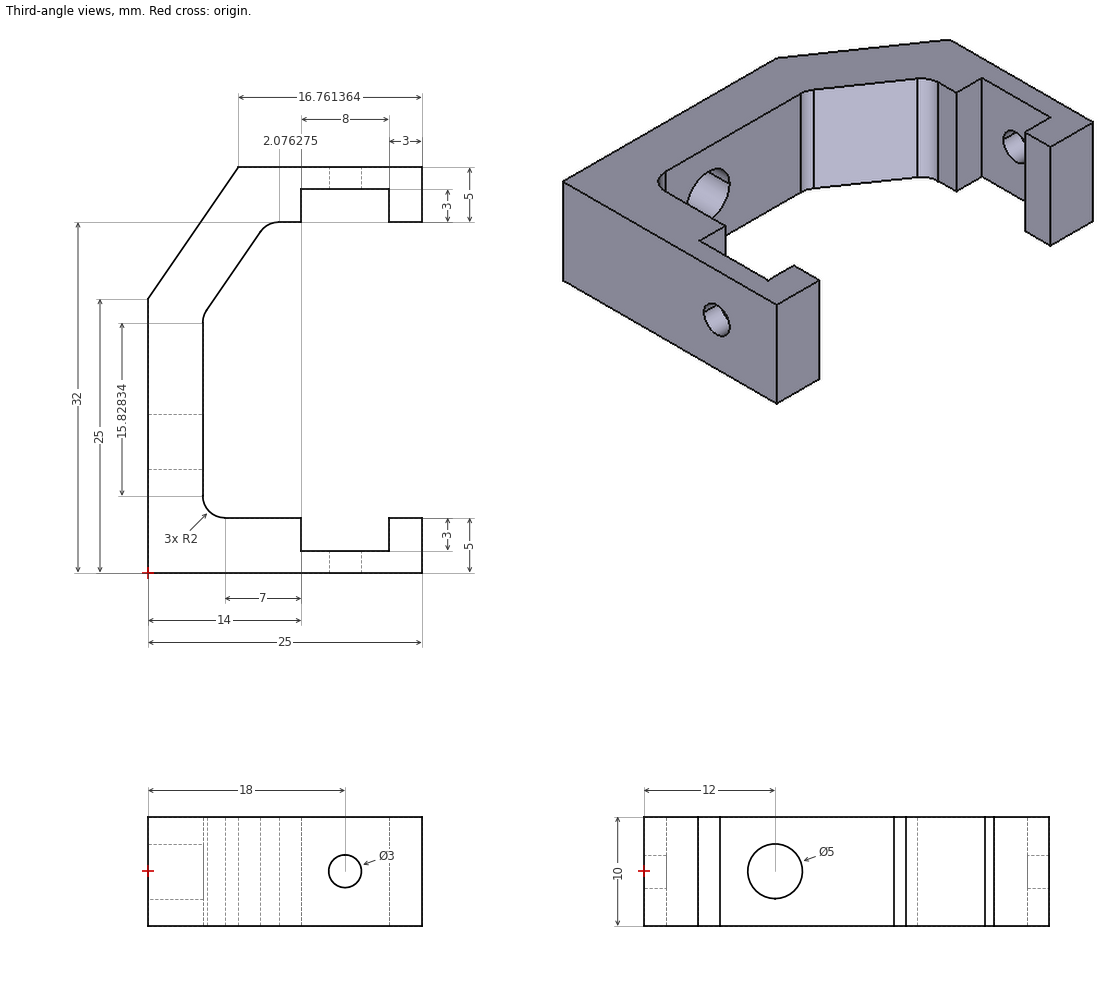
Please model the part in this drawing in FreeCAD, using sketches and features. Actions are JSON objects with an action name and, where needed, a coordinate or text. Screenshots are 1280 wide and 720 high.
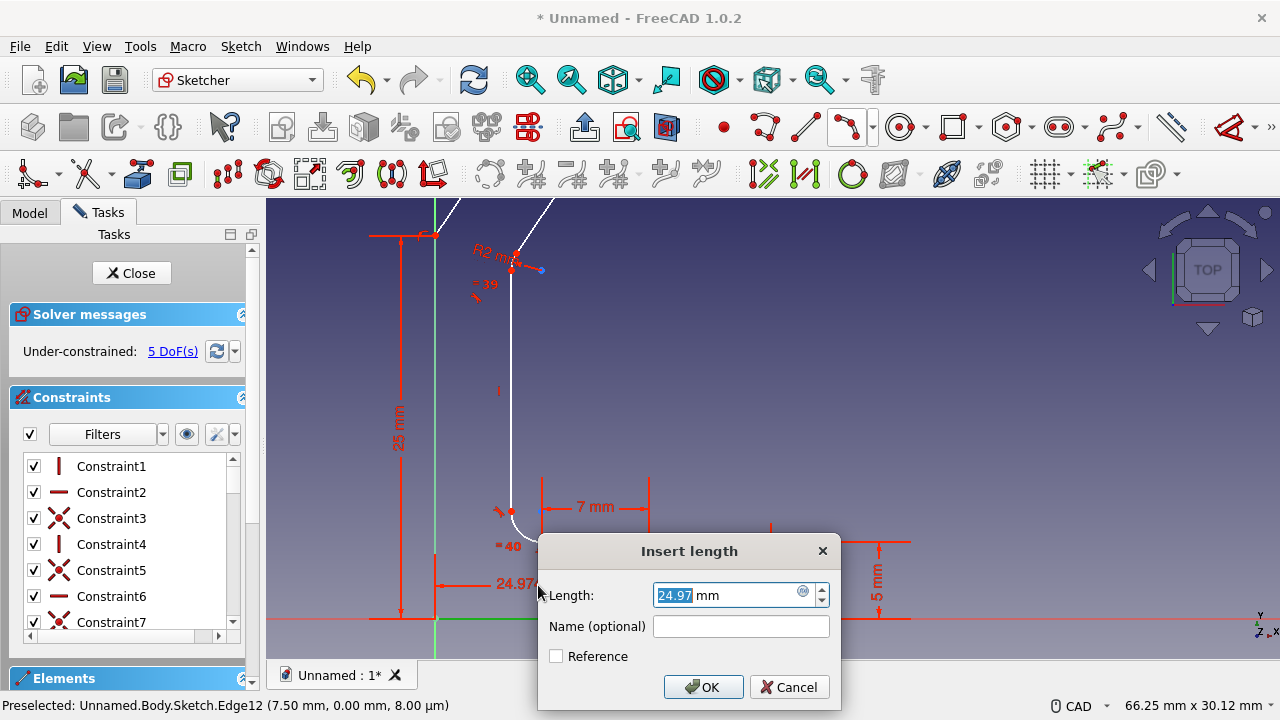
{"action": "type", "text": "25"}
{"action": "key", "text": "Return"}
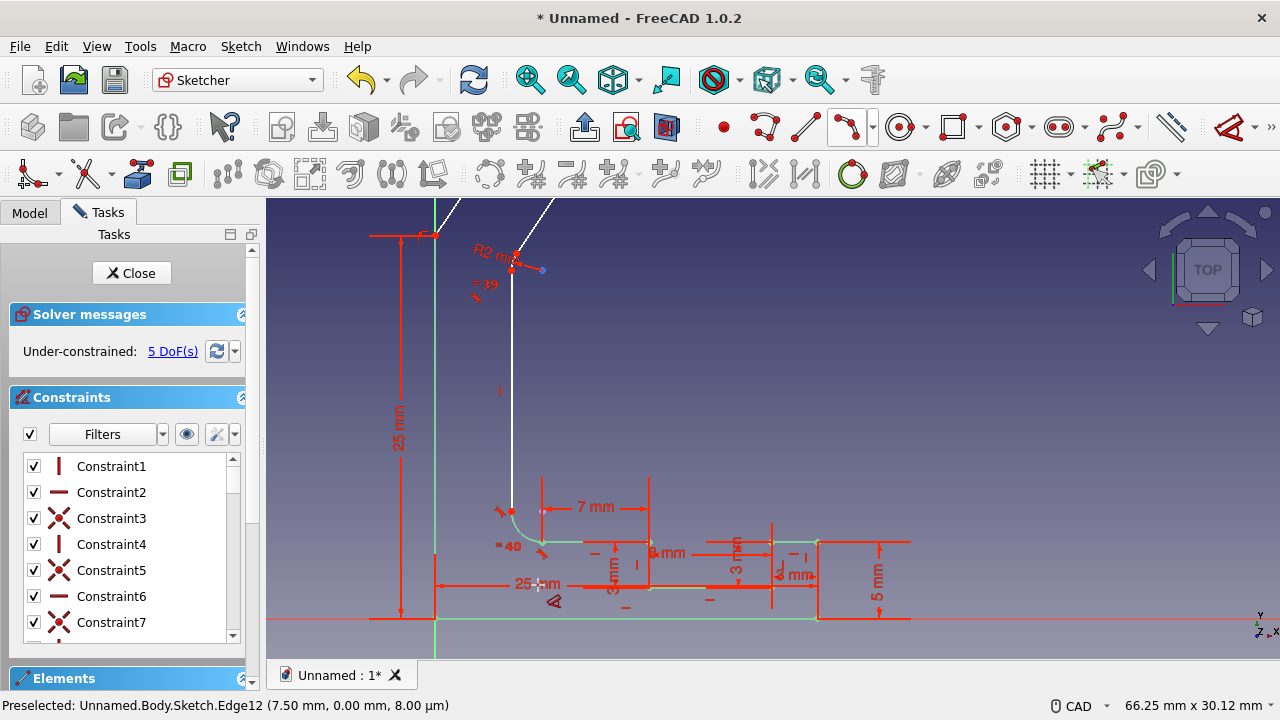
{"action": "scroll", "coordinate": [799, 542], "scroll_direction": "down", "scroll_amount": 3}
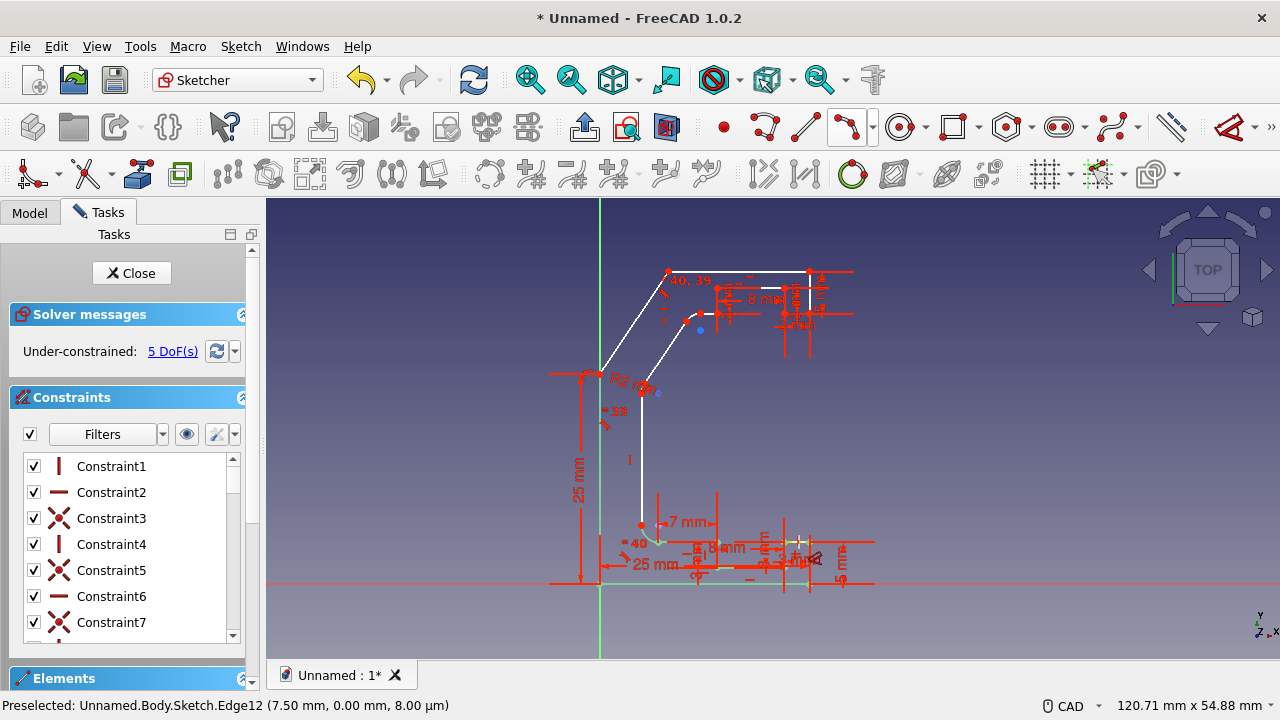
{"action": "left_click", "coordinate": [701, 314]}
{"action": "left_click", "coordinate": [566, 449]}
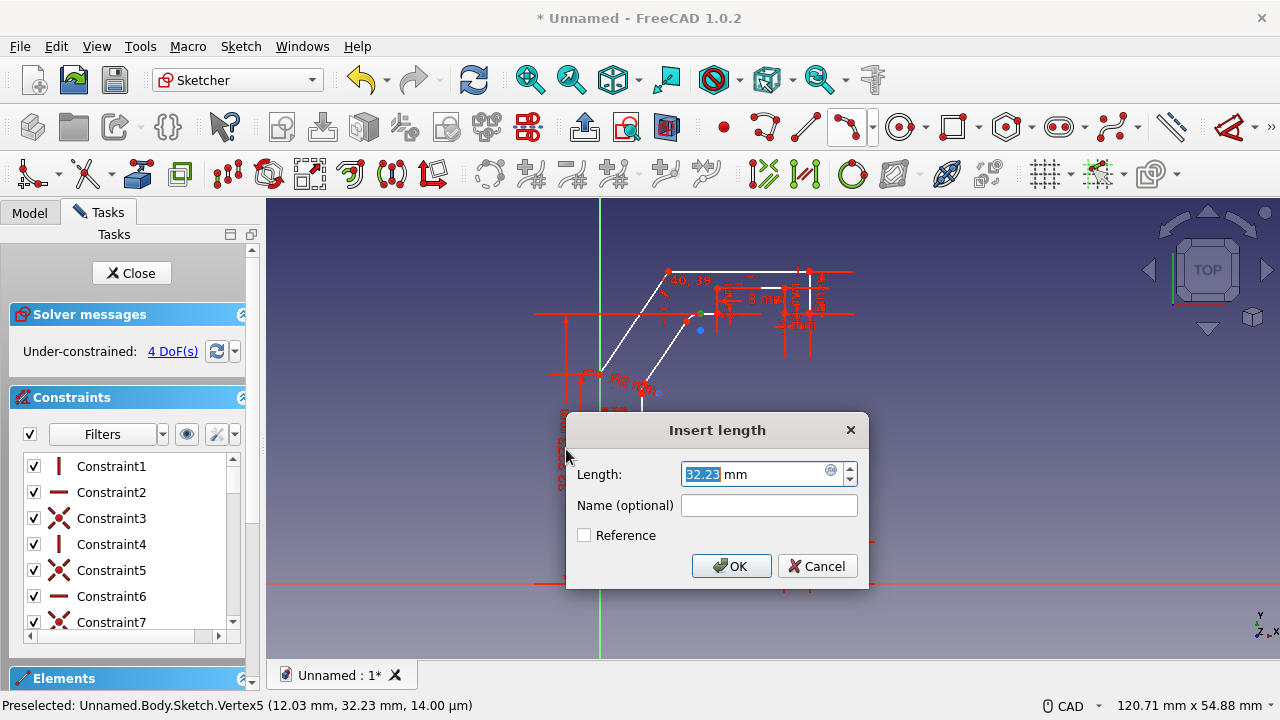
{"action": "type", "text": "32"}
{"action": "key", "text": "Return"}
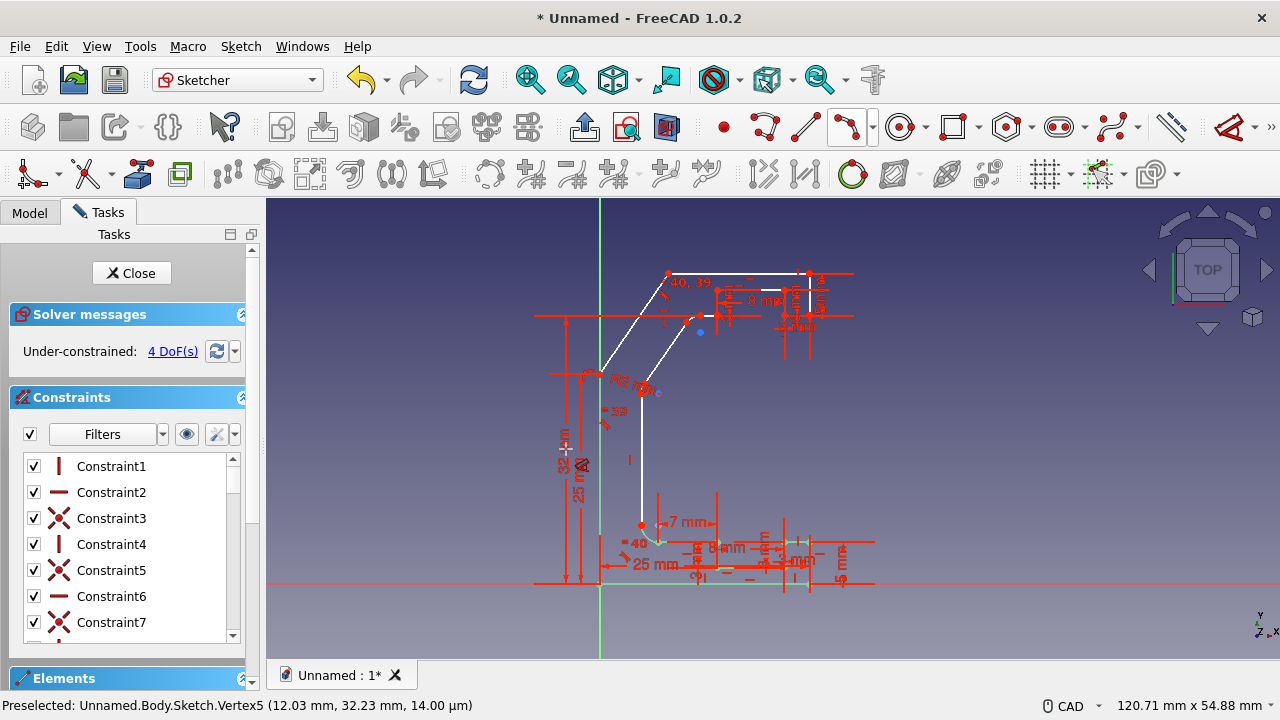
{"action": "left_click", "coordinate": [717, 316]}
{"action": "left_click", "coordinate": [658, 618]}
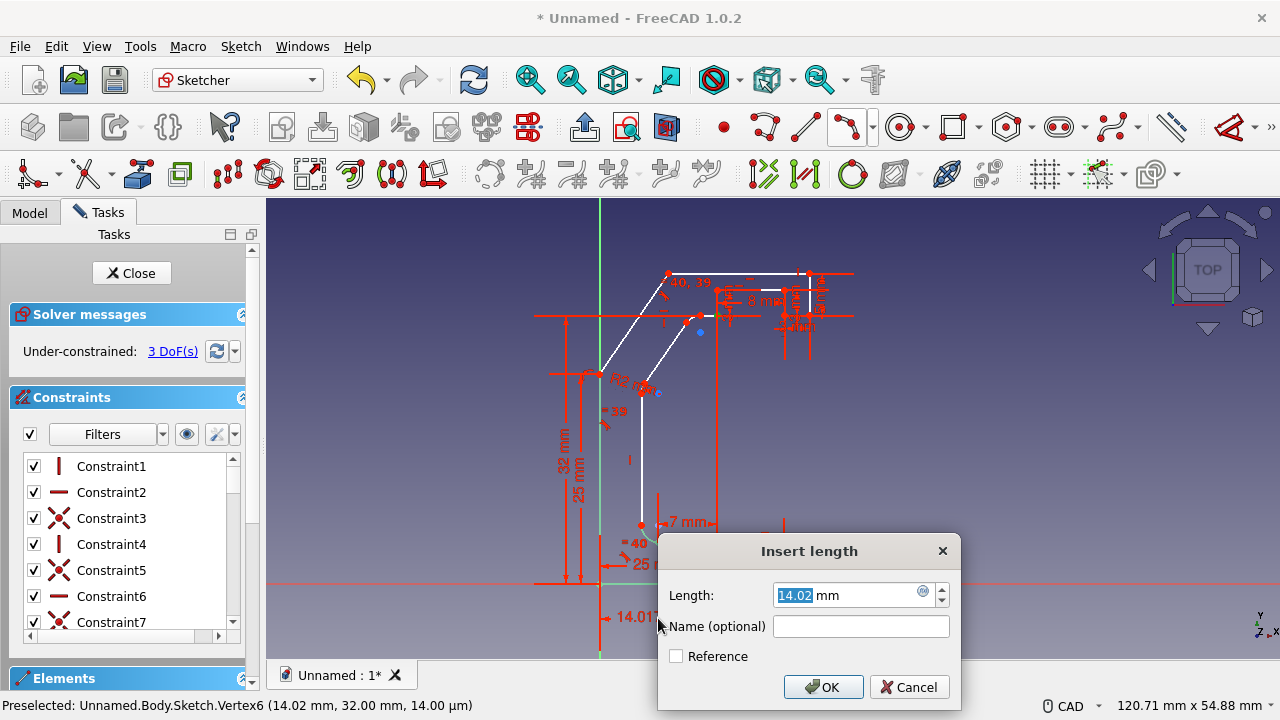
{"action": "type", "text": "14"}
{"action": "key", "text": "Return"}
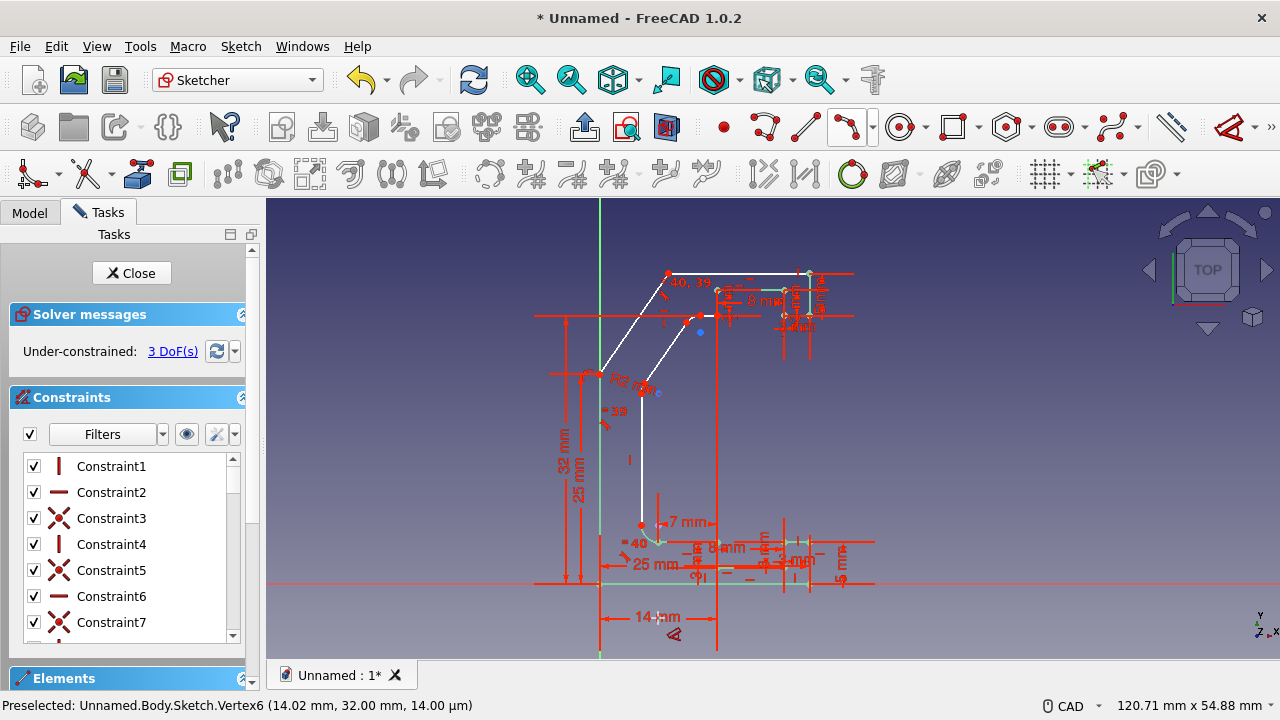
{"action": "left_click", "coordinate": [642, 486]}
{"action": "left_click", "coordinate": [676, 460]}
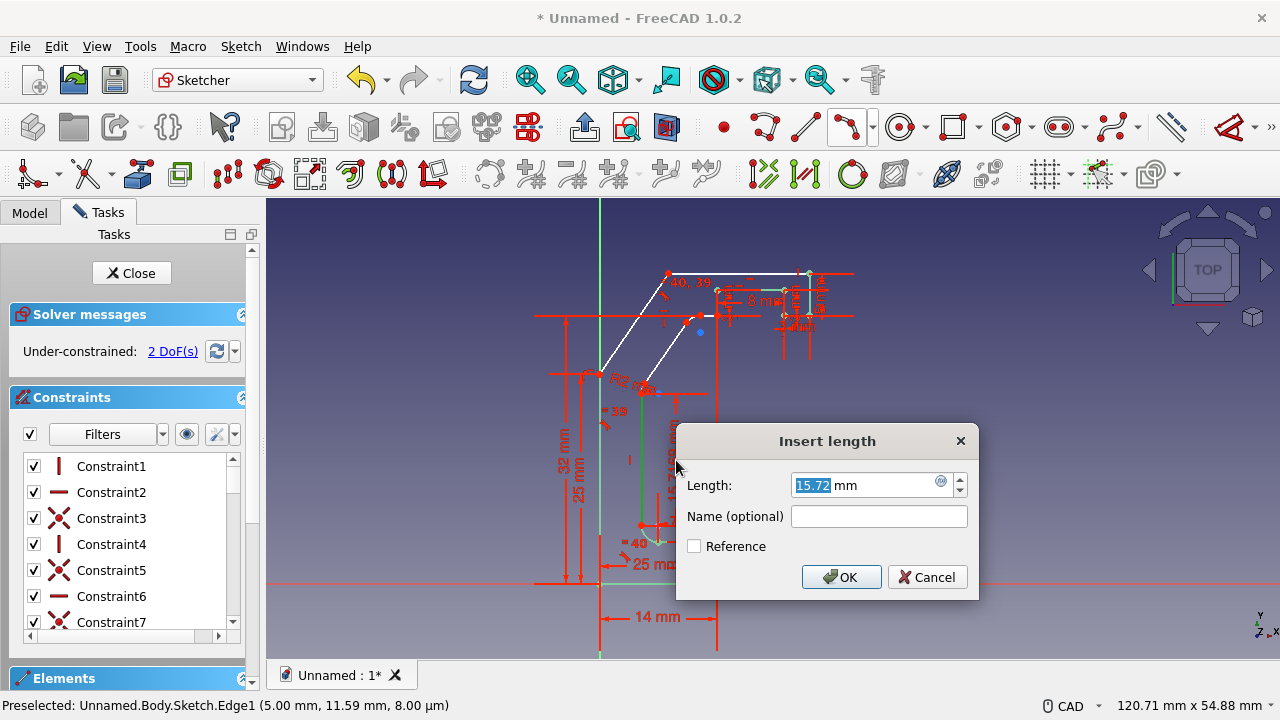
{"action": "type", "text": "15.82834"}
{"action": "key", "text": "Return"}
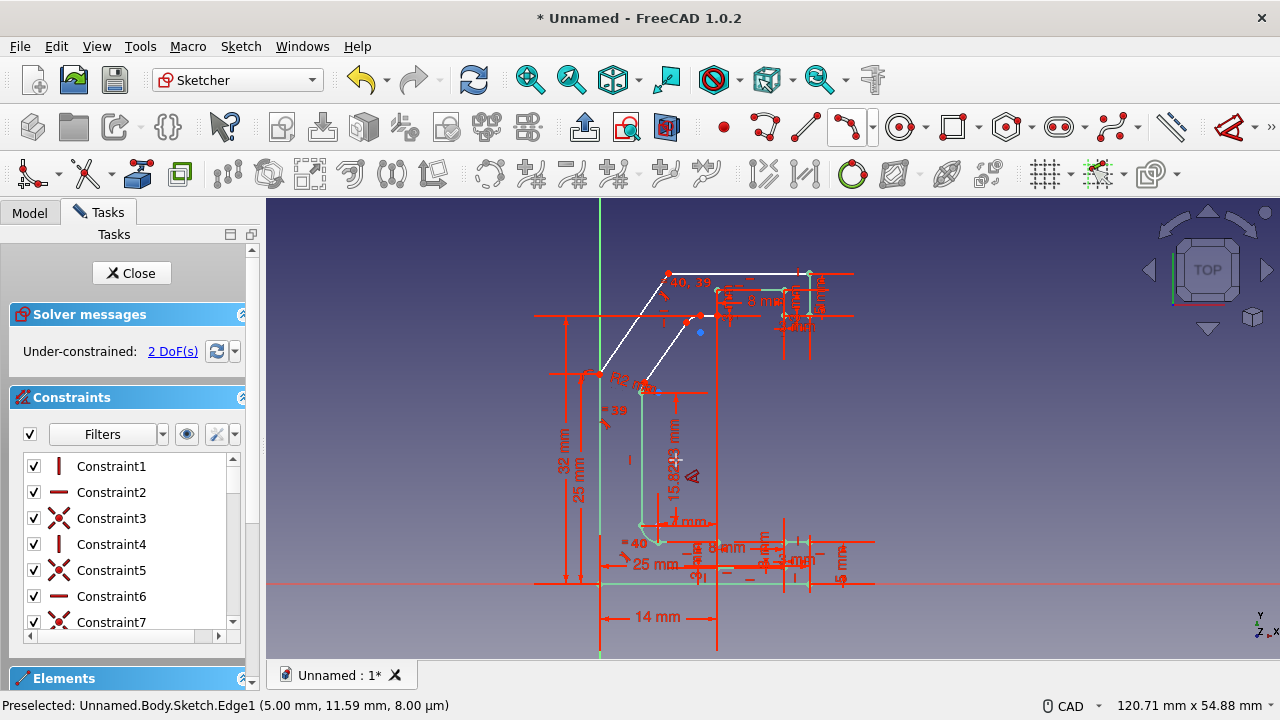
{"action": "scroll", "coordinate": [709, 316], "scroll_direction": "up", "scroll_amount": 5}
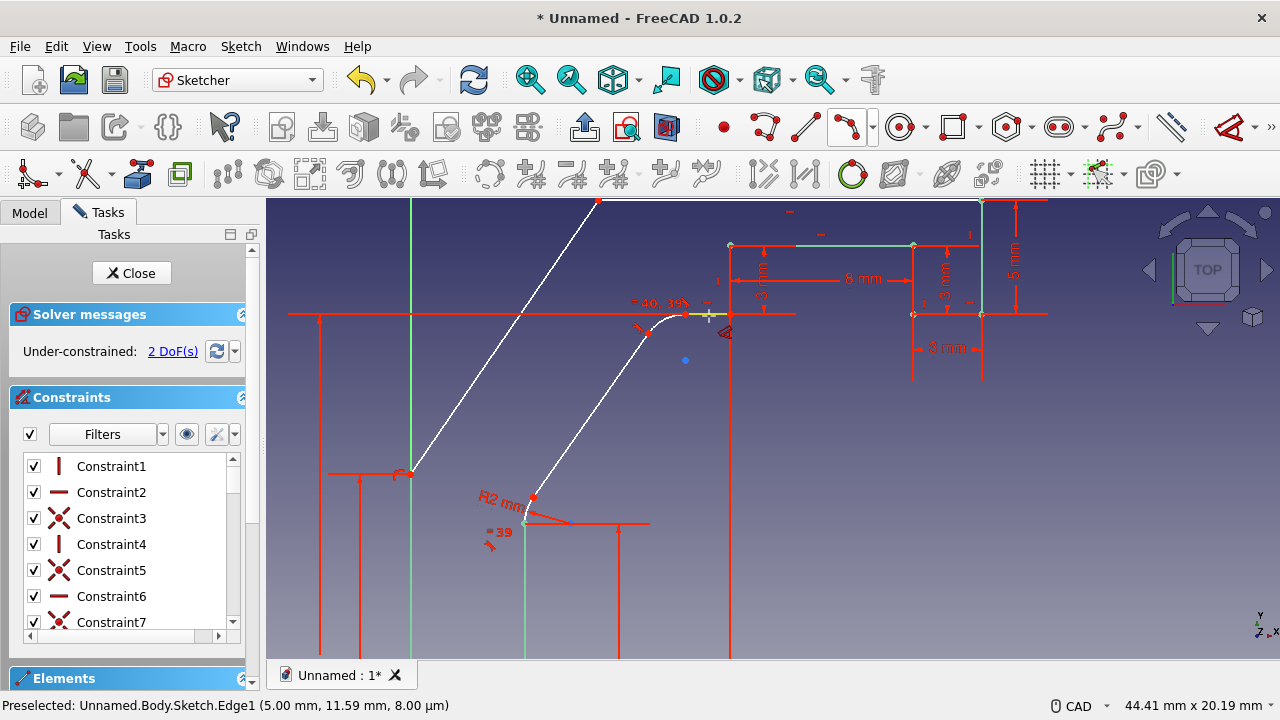
{"action": "left_click", "coordinate": [708, 314]}
{"action": "left_click", "coordinate": [692, 280]}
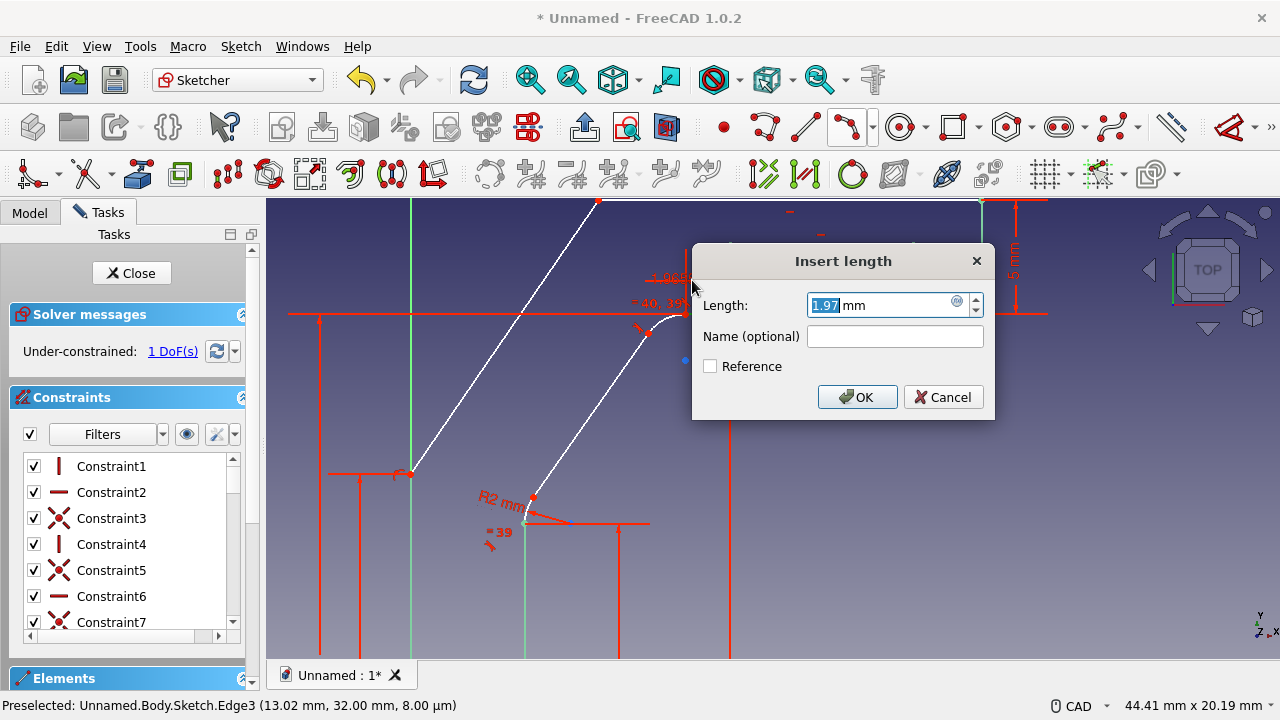
{"action": "type", "text": "2.076275"}
{"action": "key", "text": "Return"}